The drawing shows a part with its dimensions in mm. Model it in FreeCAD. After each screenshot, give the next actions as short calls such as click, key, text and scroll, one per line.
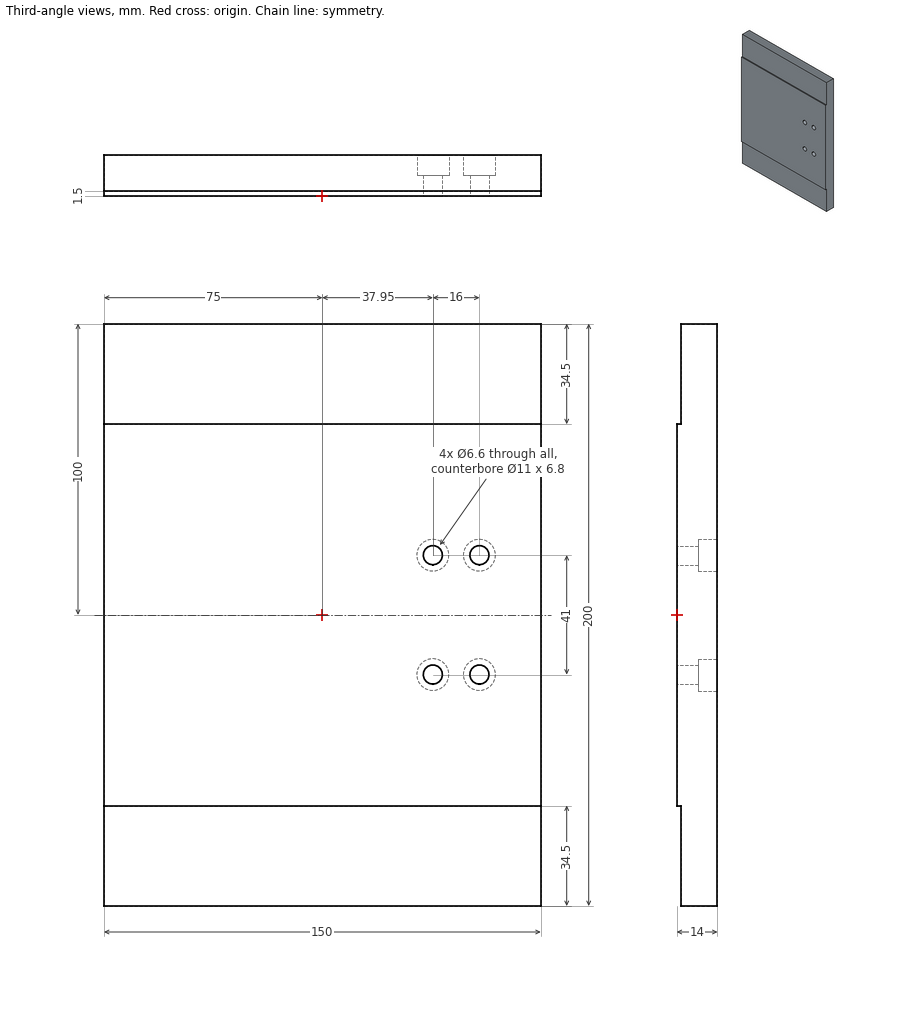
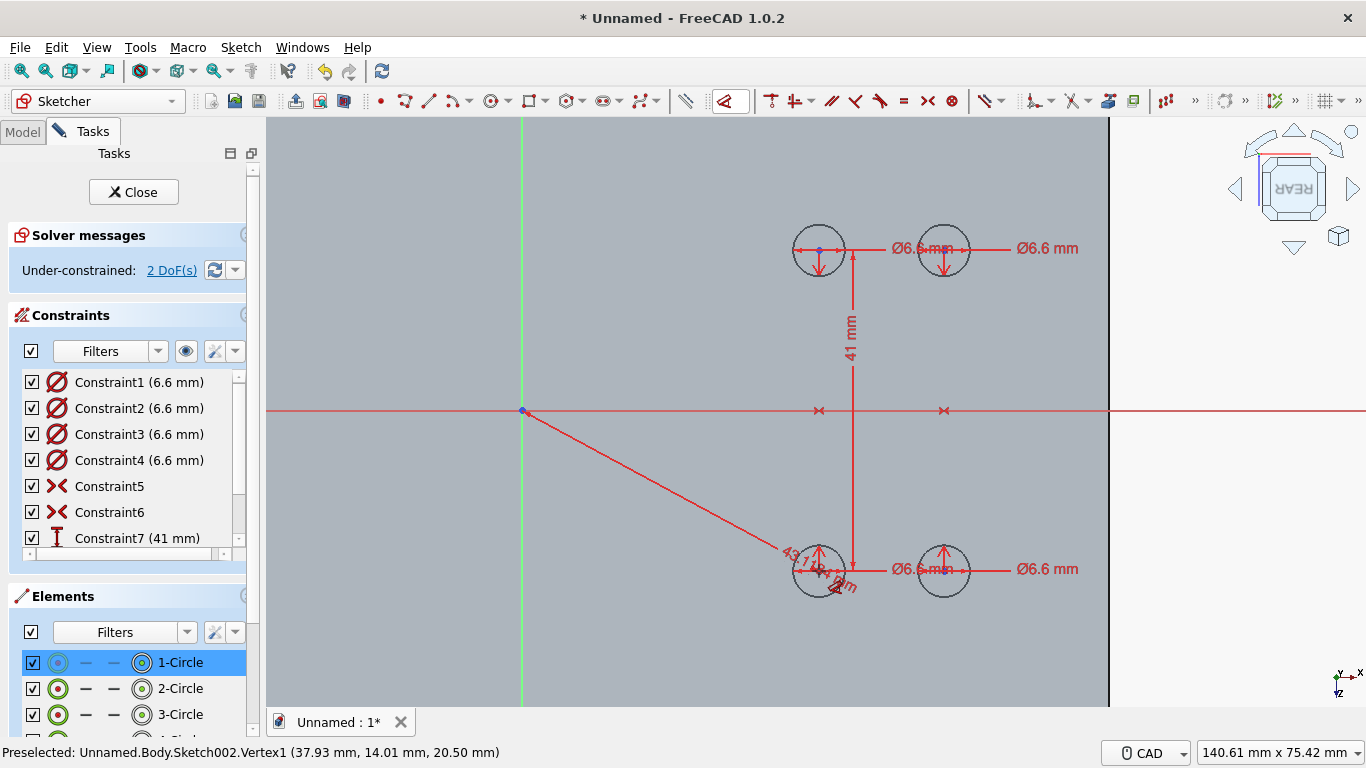
click(944, 571)
click(882, 605)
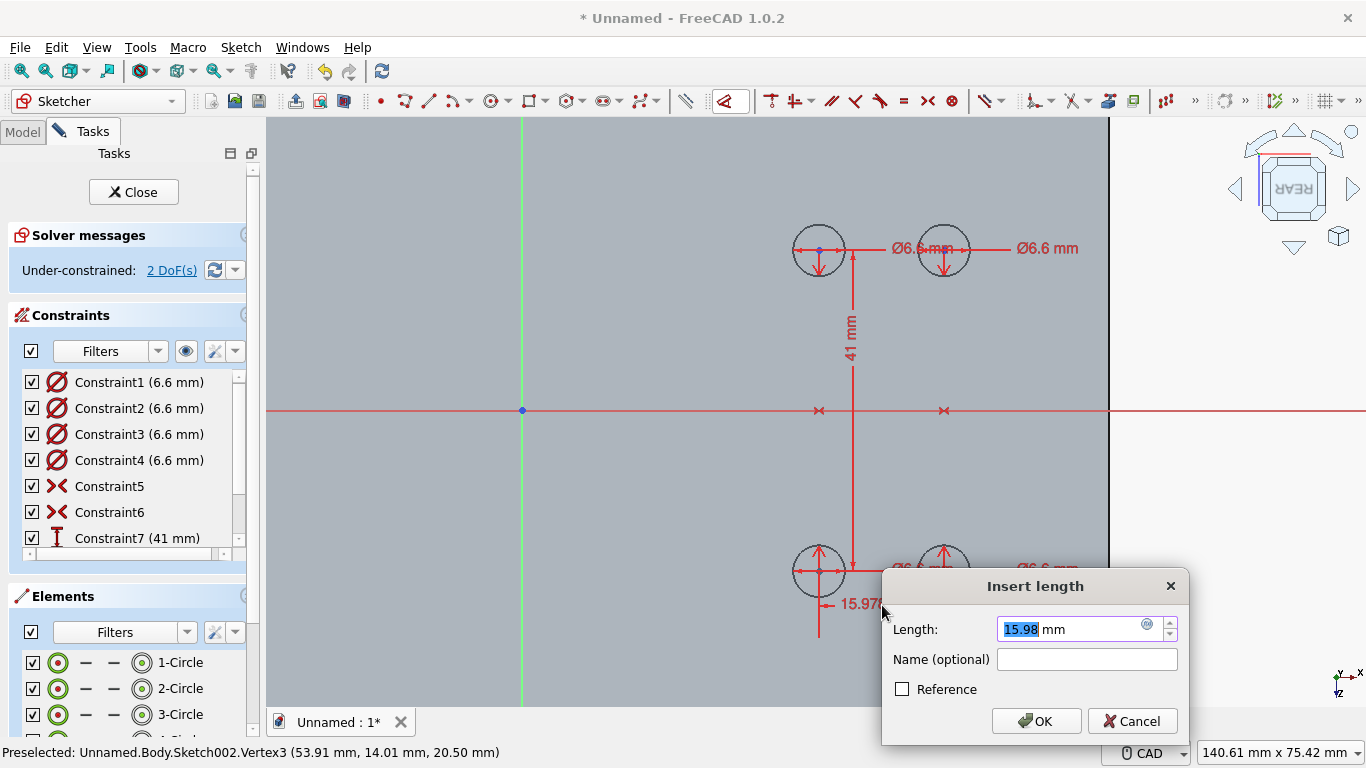
text(16)
key(Return)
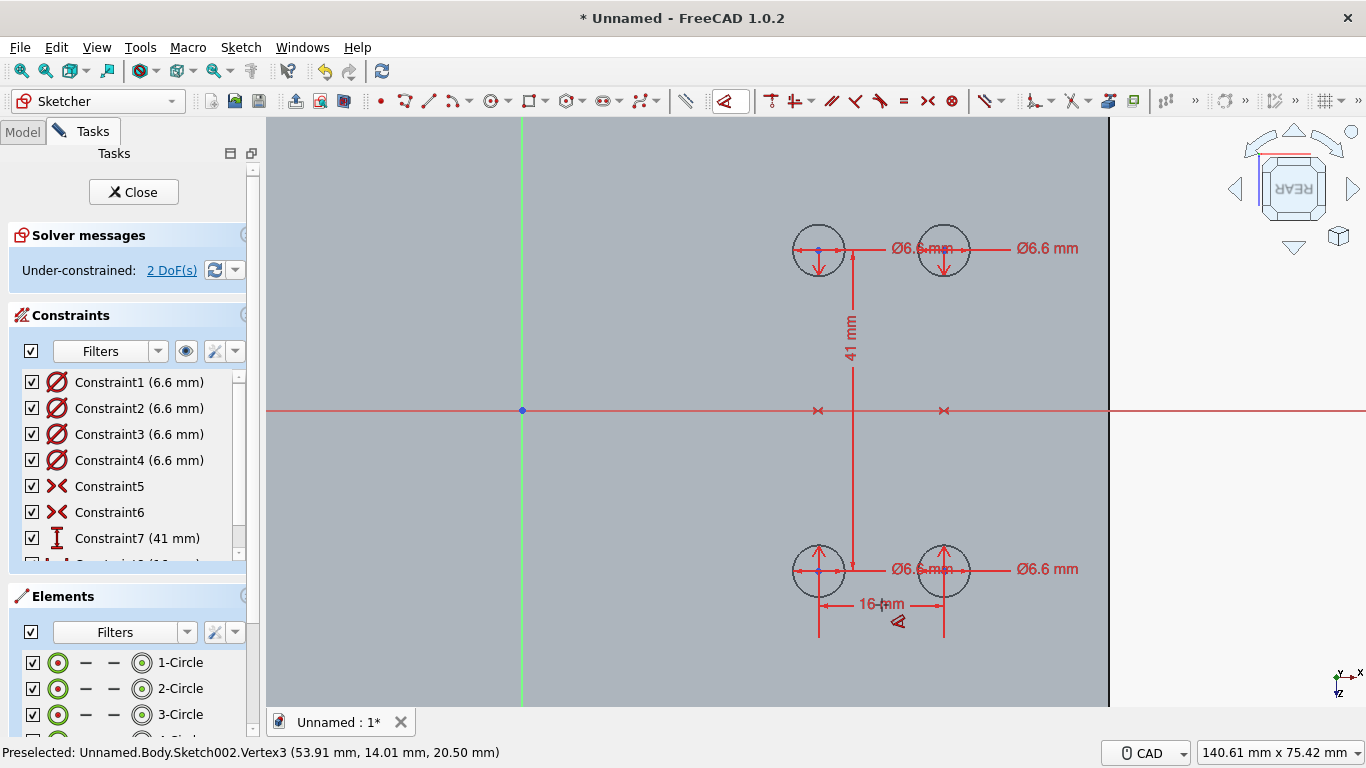
click(819, 250)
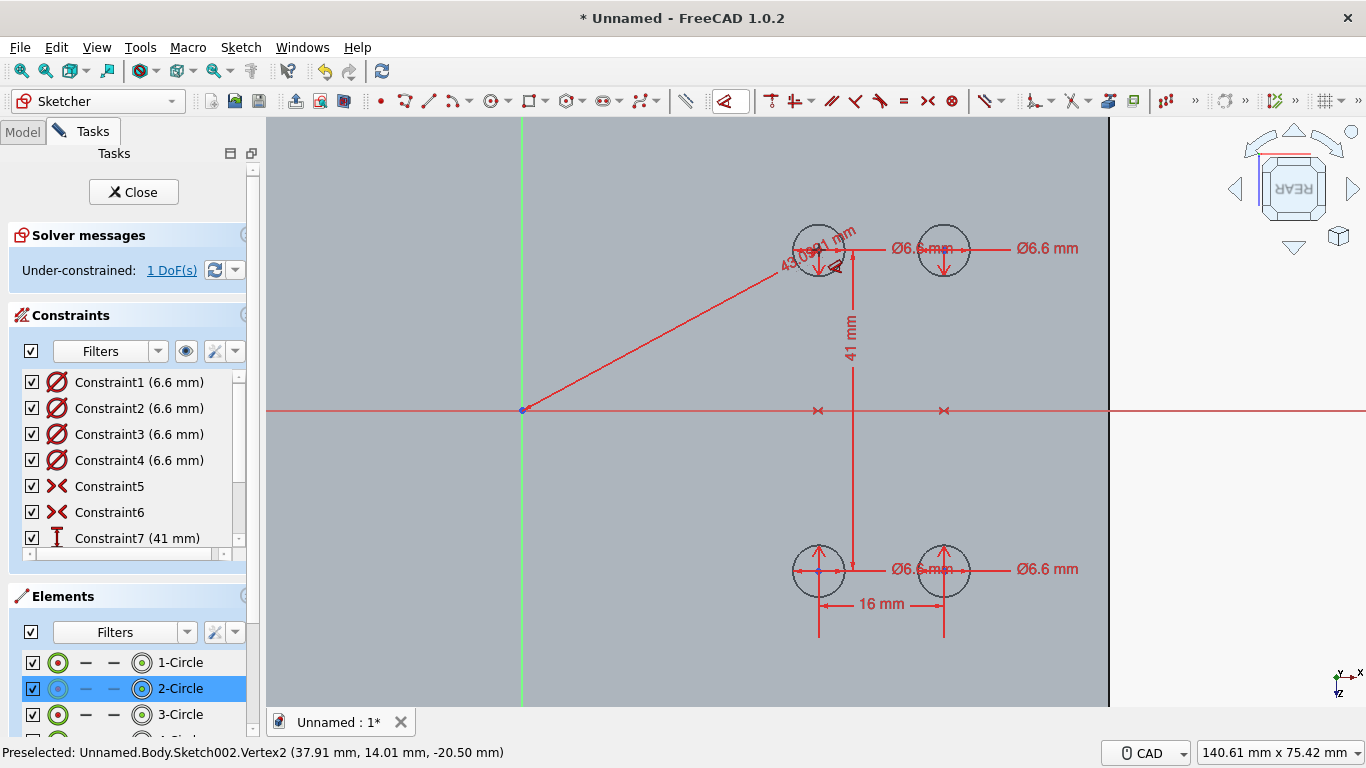
click(944, 571)
click(978, 337)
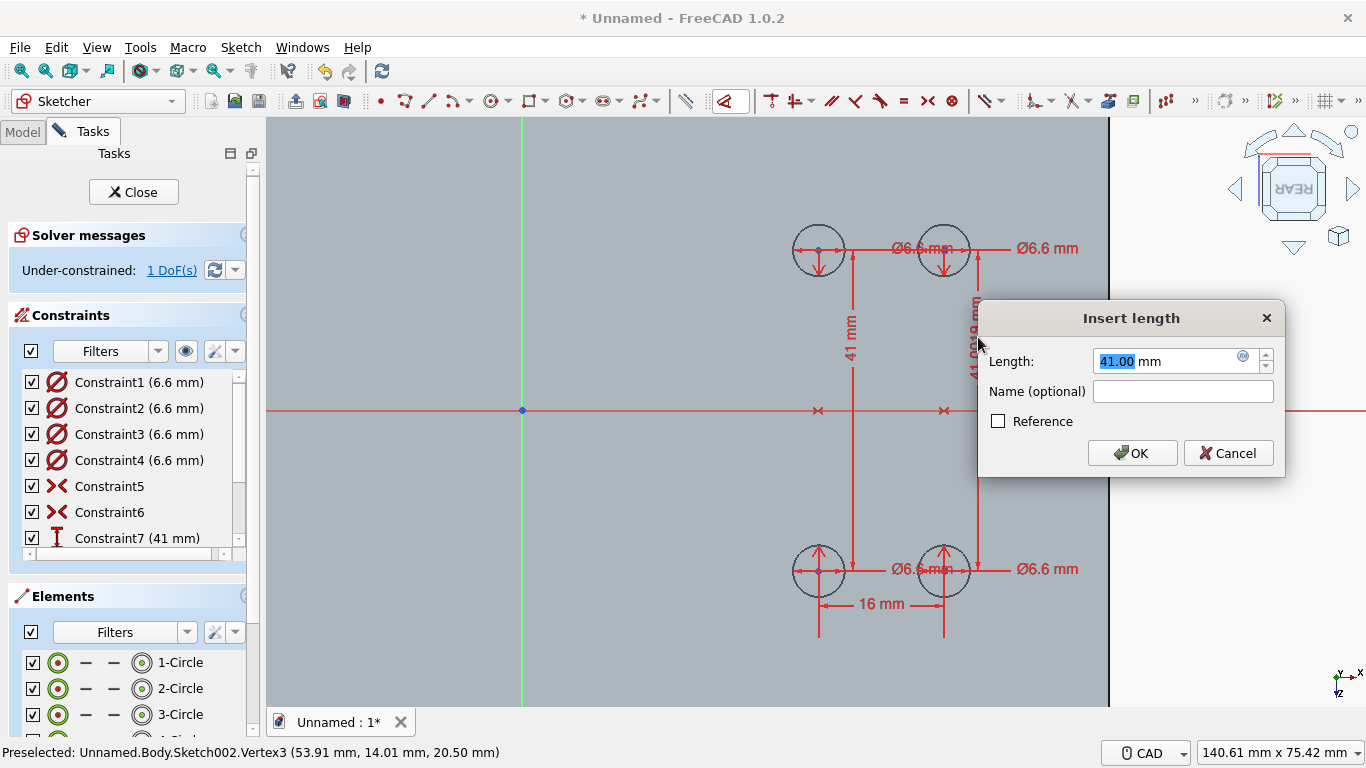
text(41)
key(Return)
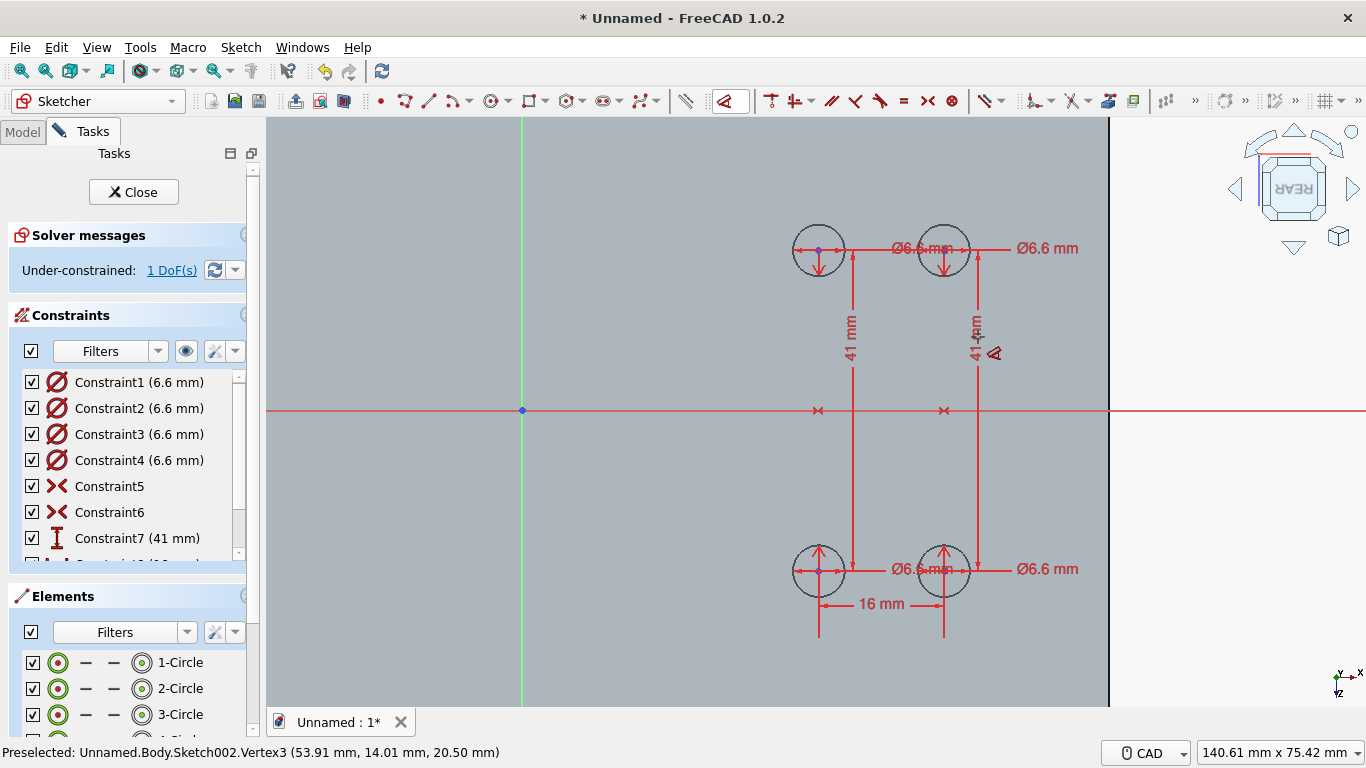
click(819, 571)
click(671, 605)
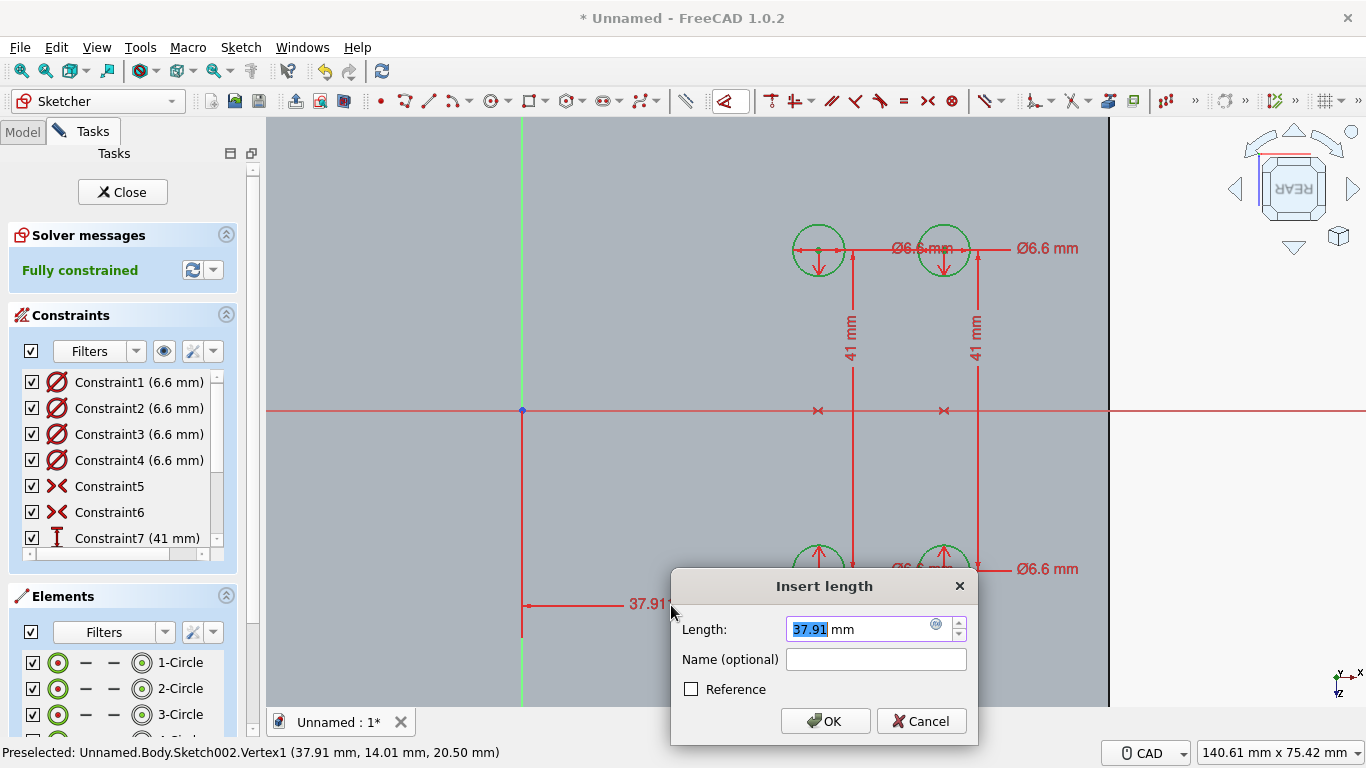
text(37.95)
key(Return)
key(Escape)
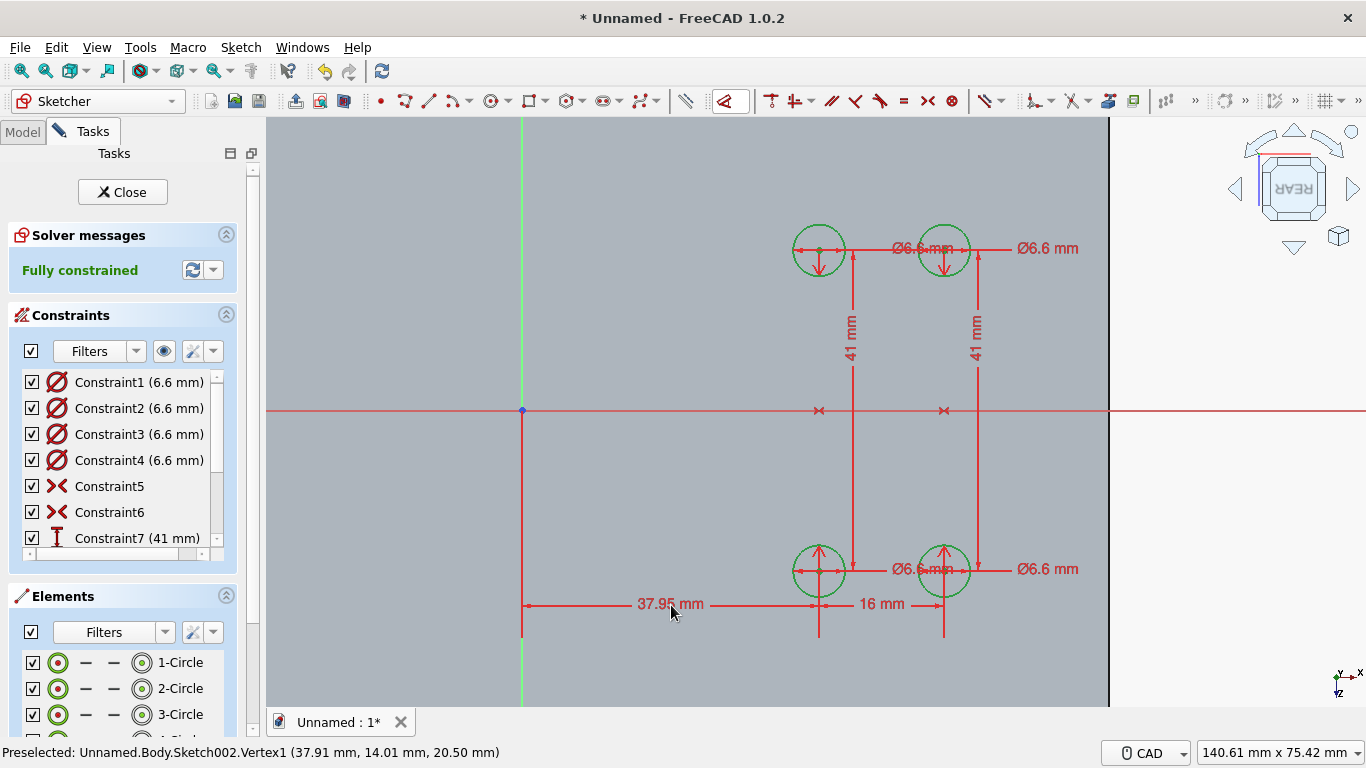
click(123, 192)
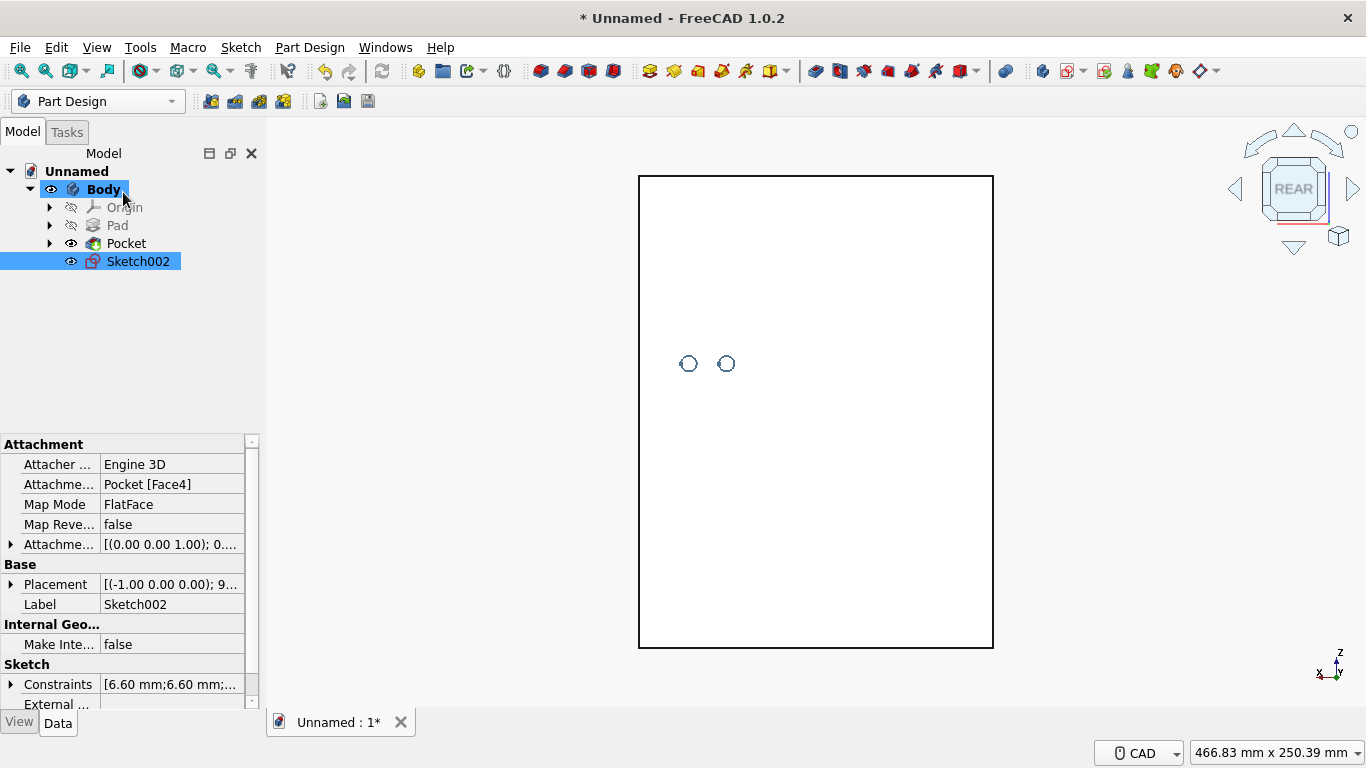
click(840, 72)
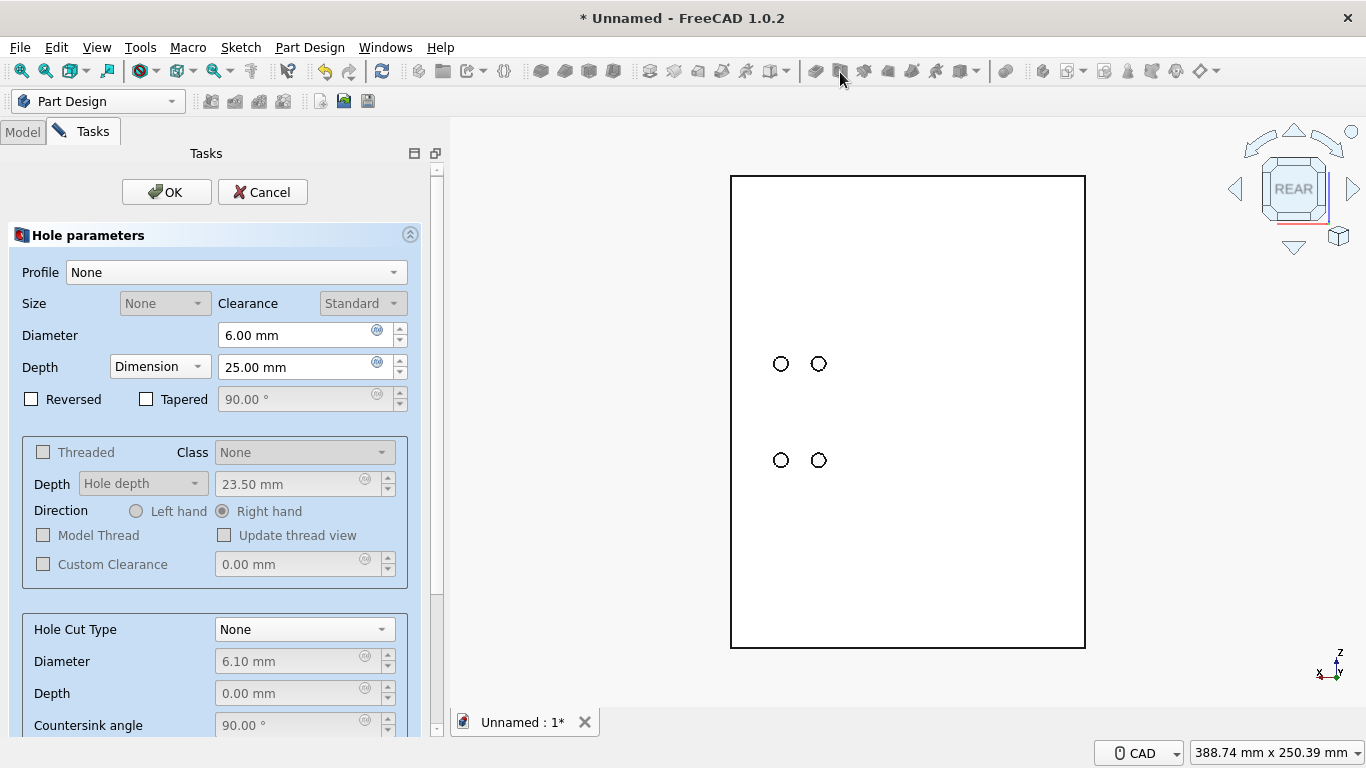
triple_click(305, 335)